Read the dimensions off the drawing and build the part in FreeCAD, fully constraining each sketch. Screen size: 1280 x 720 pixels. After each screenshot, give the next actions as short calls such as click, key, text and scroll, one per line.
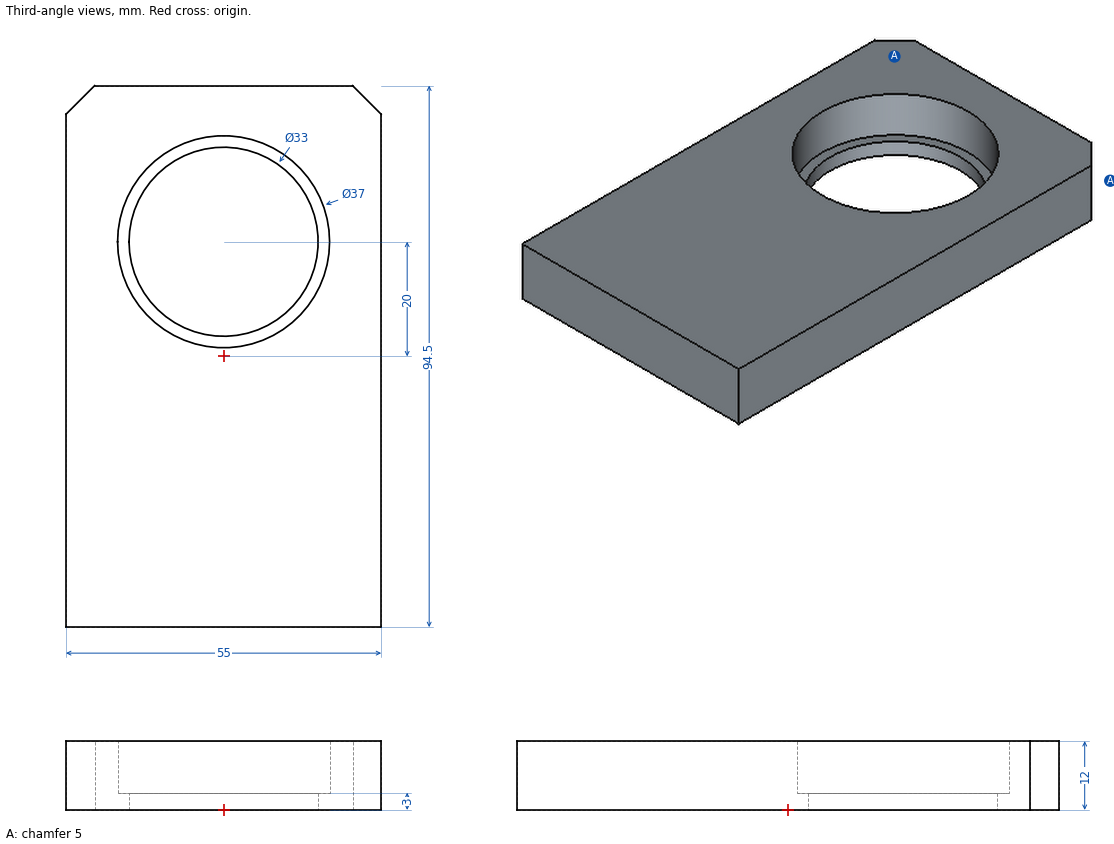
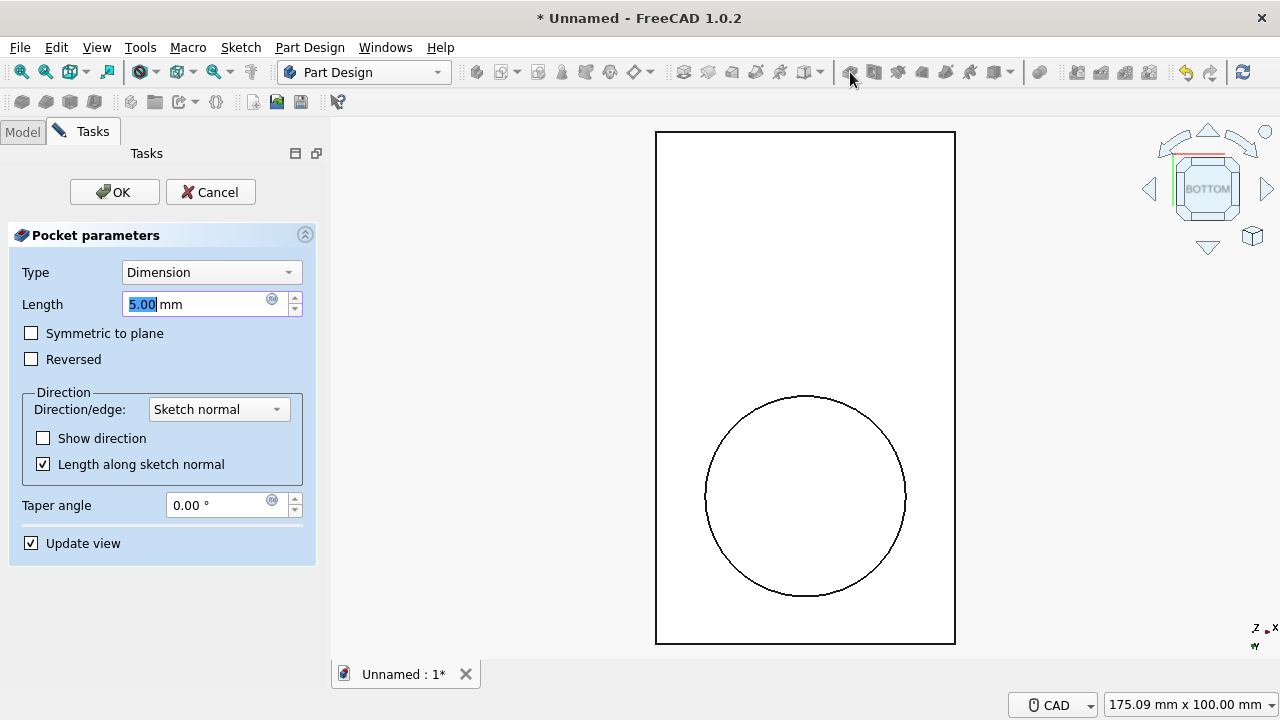
click(212, 272)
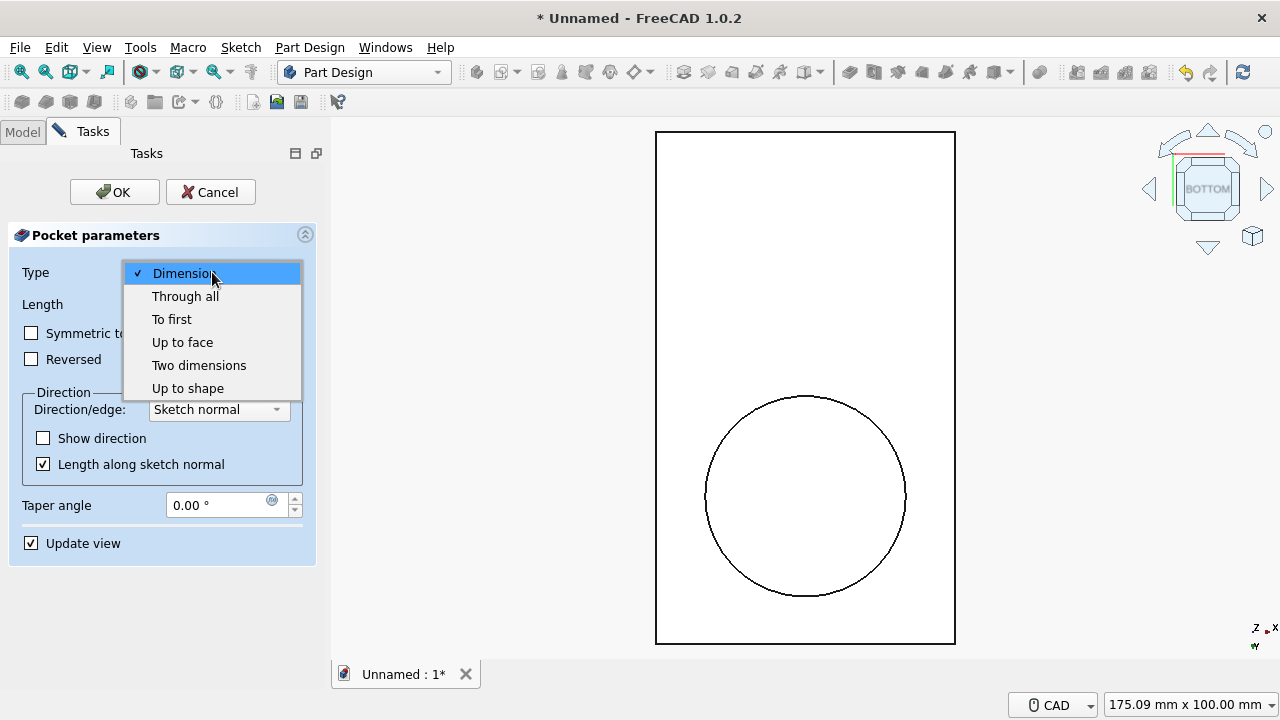
click(212, 320)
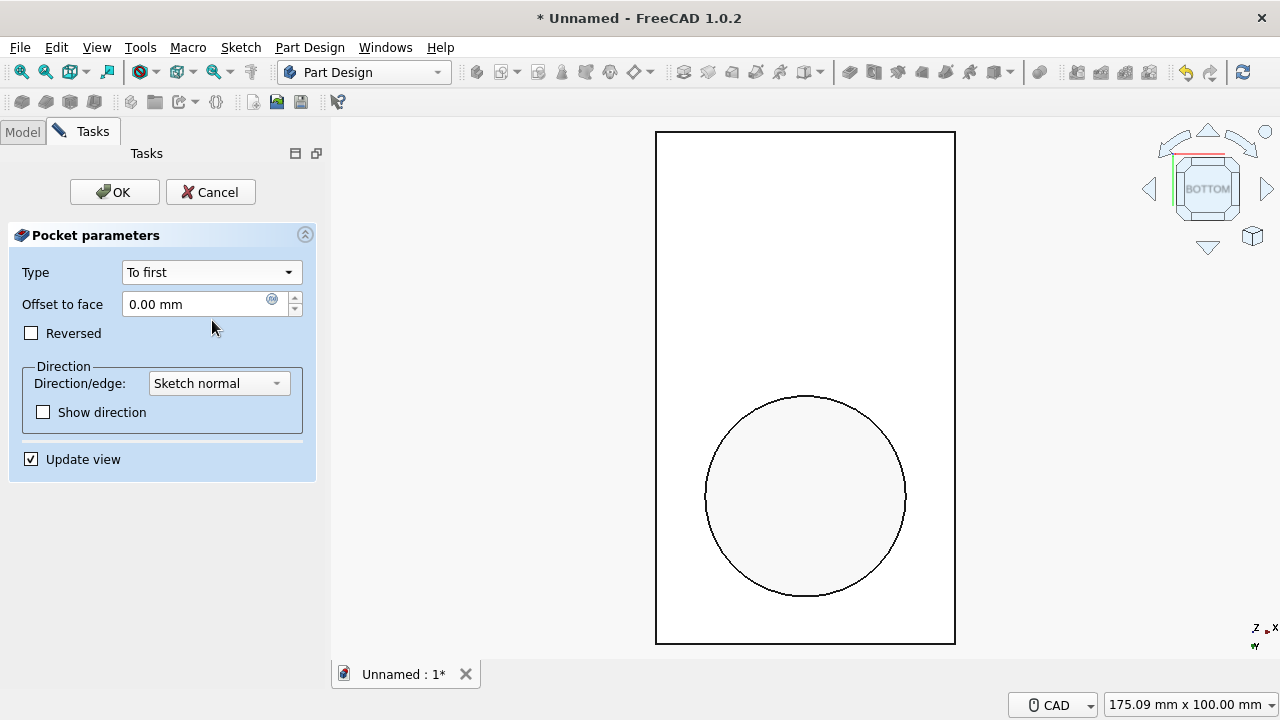
click(115, 192)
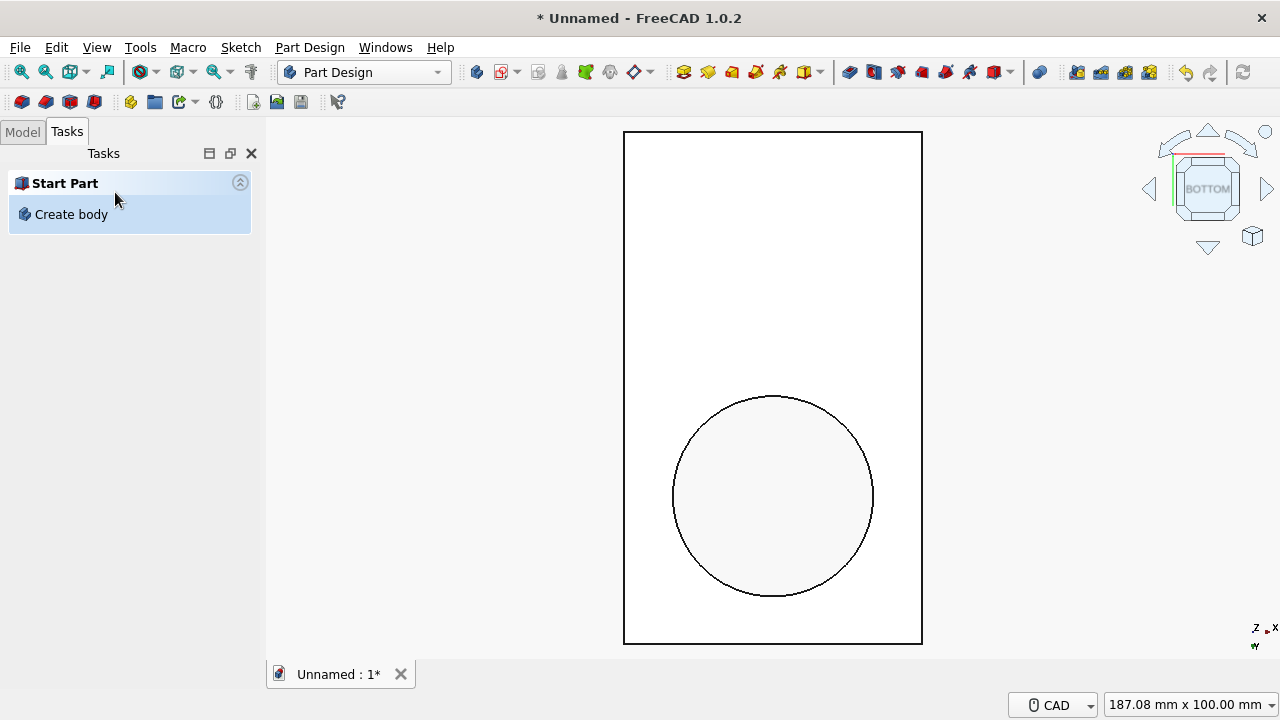
key(0)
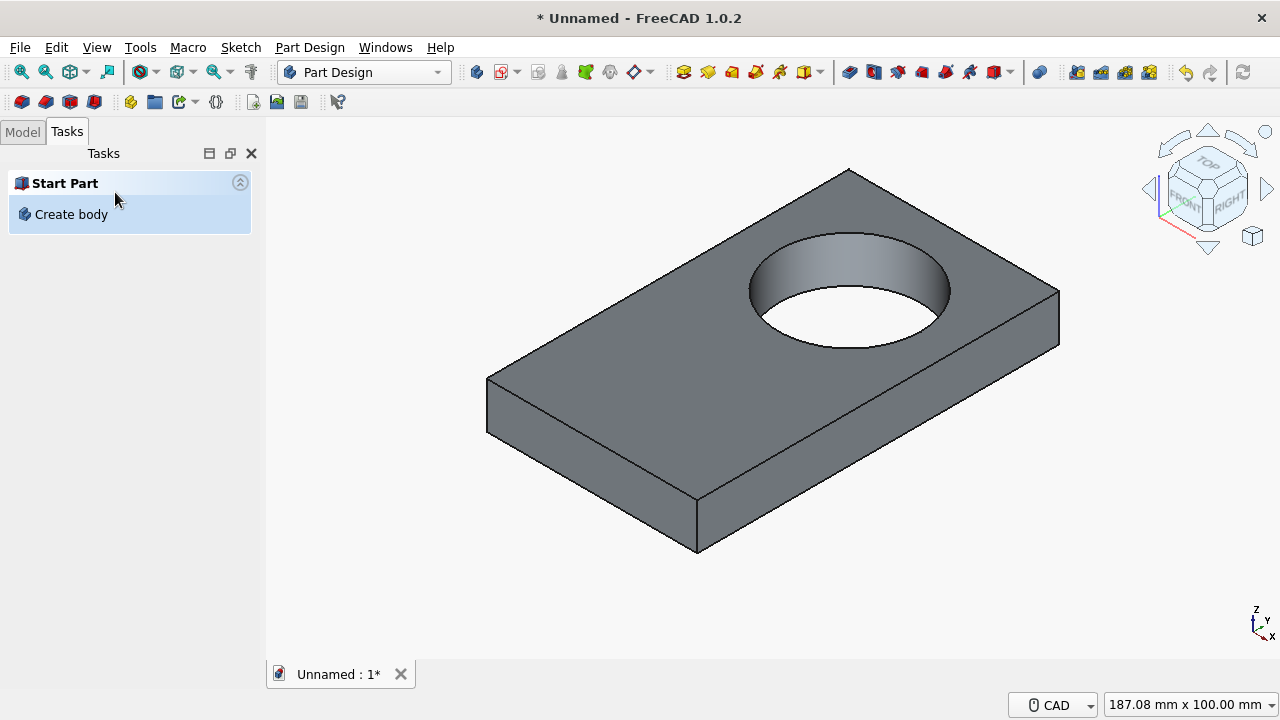
key(2)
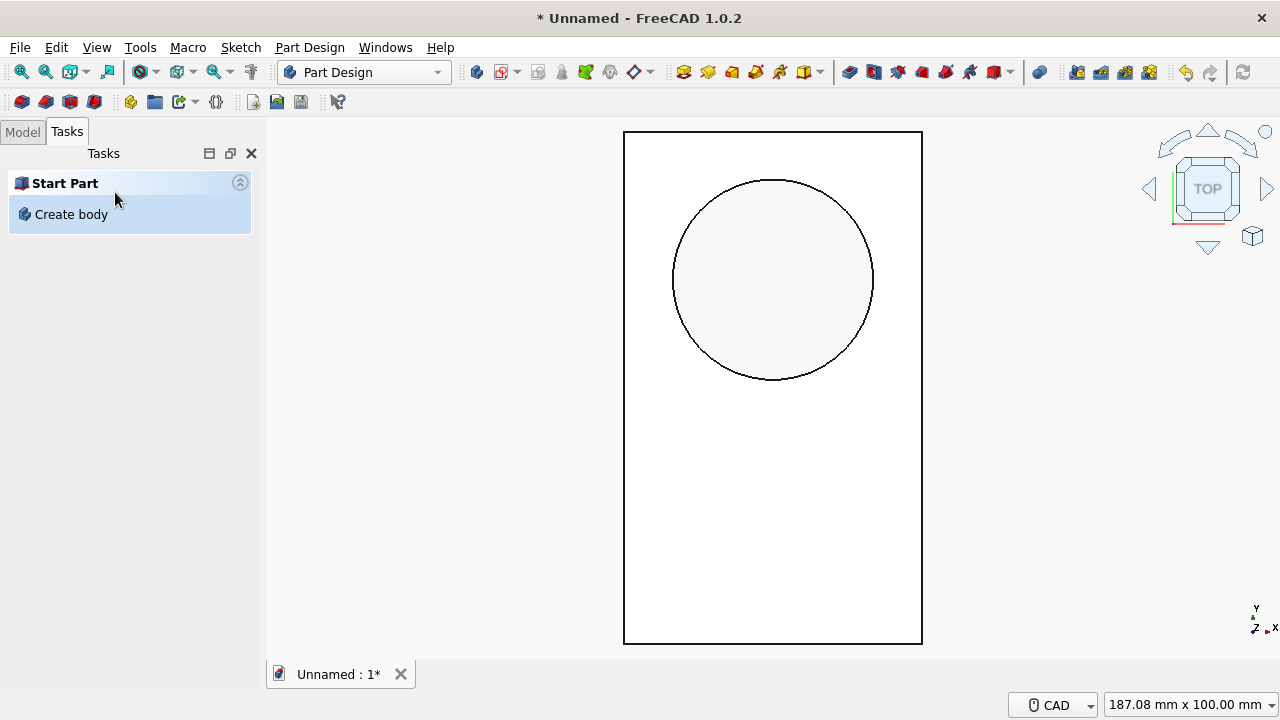
key(1)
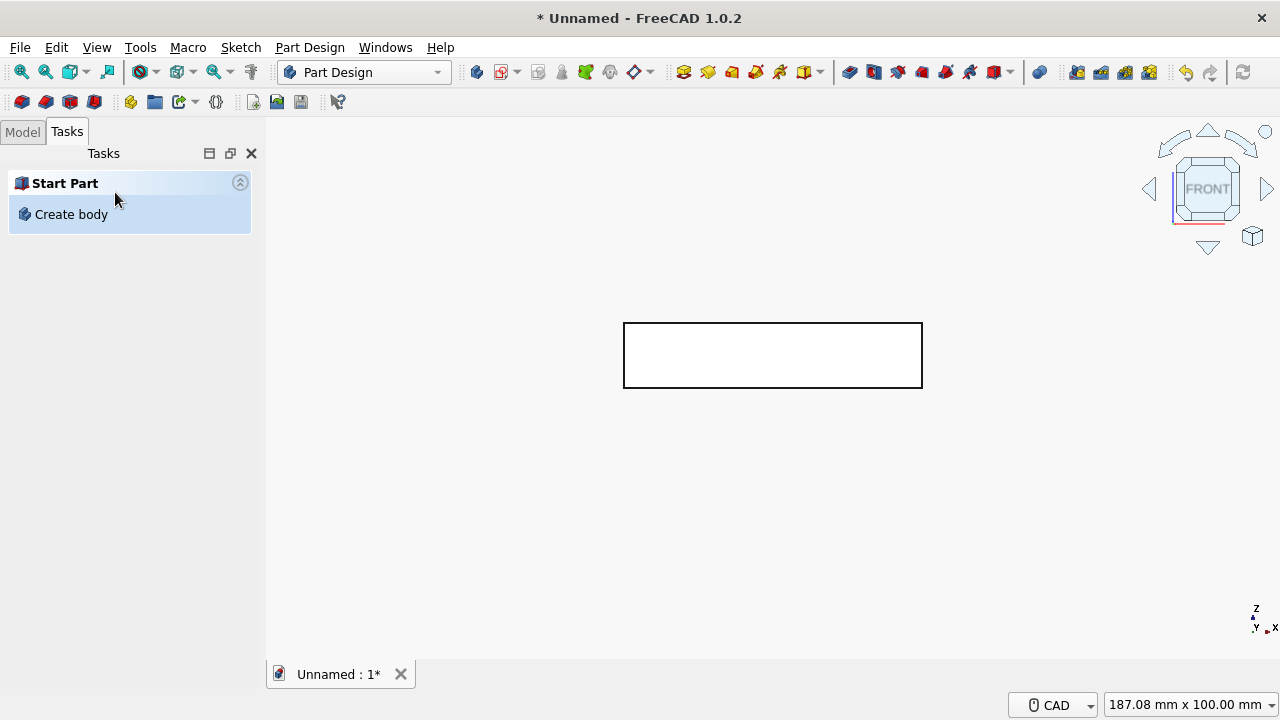
click(22, 72)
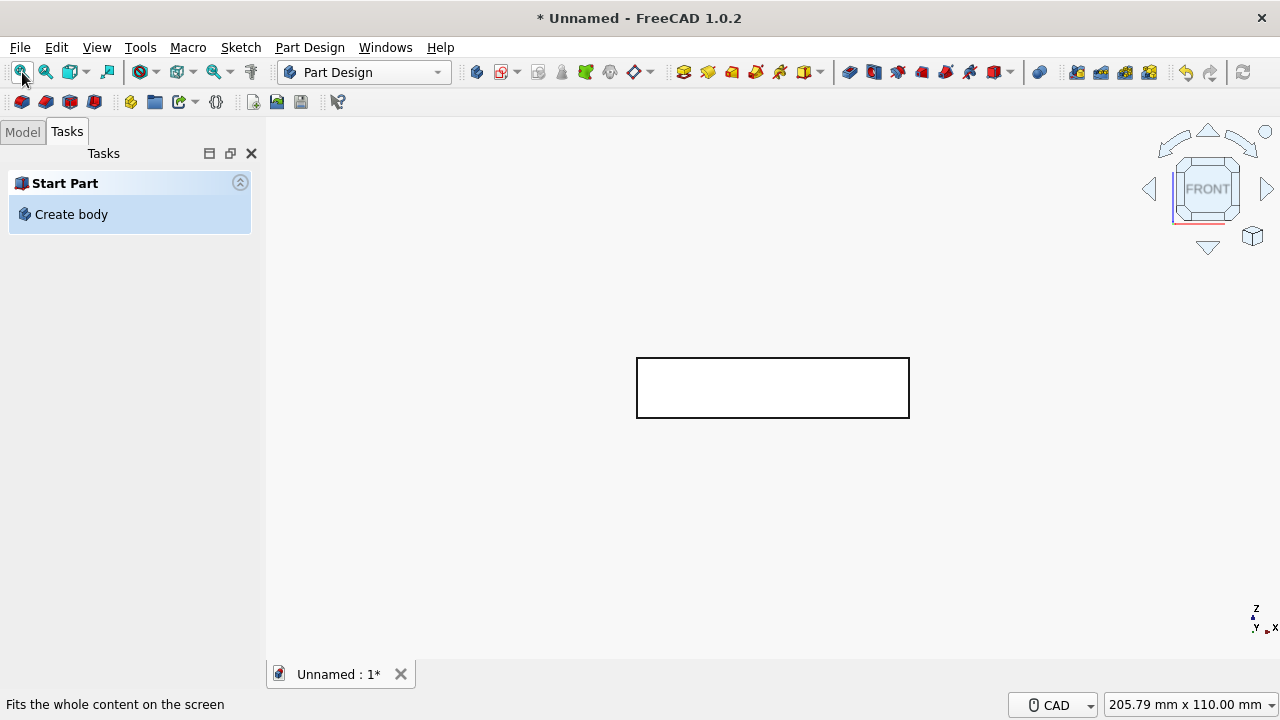
key(3)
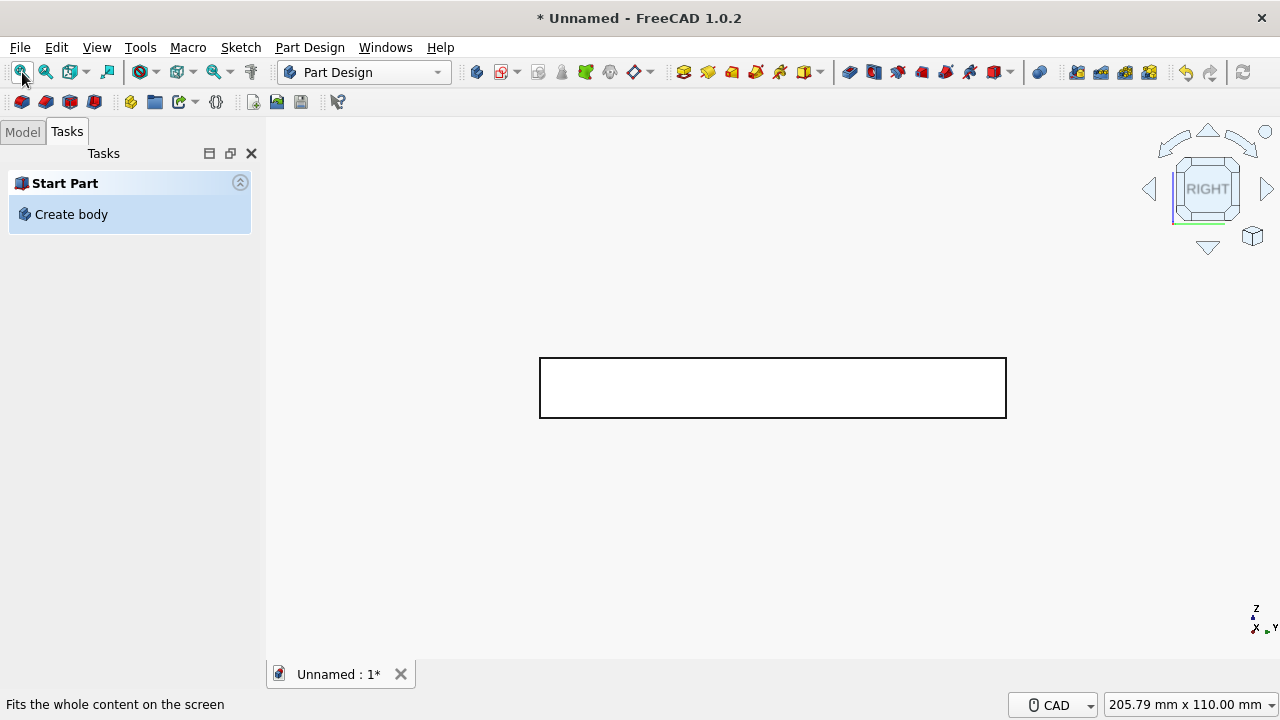
click(1006, 387)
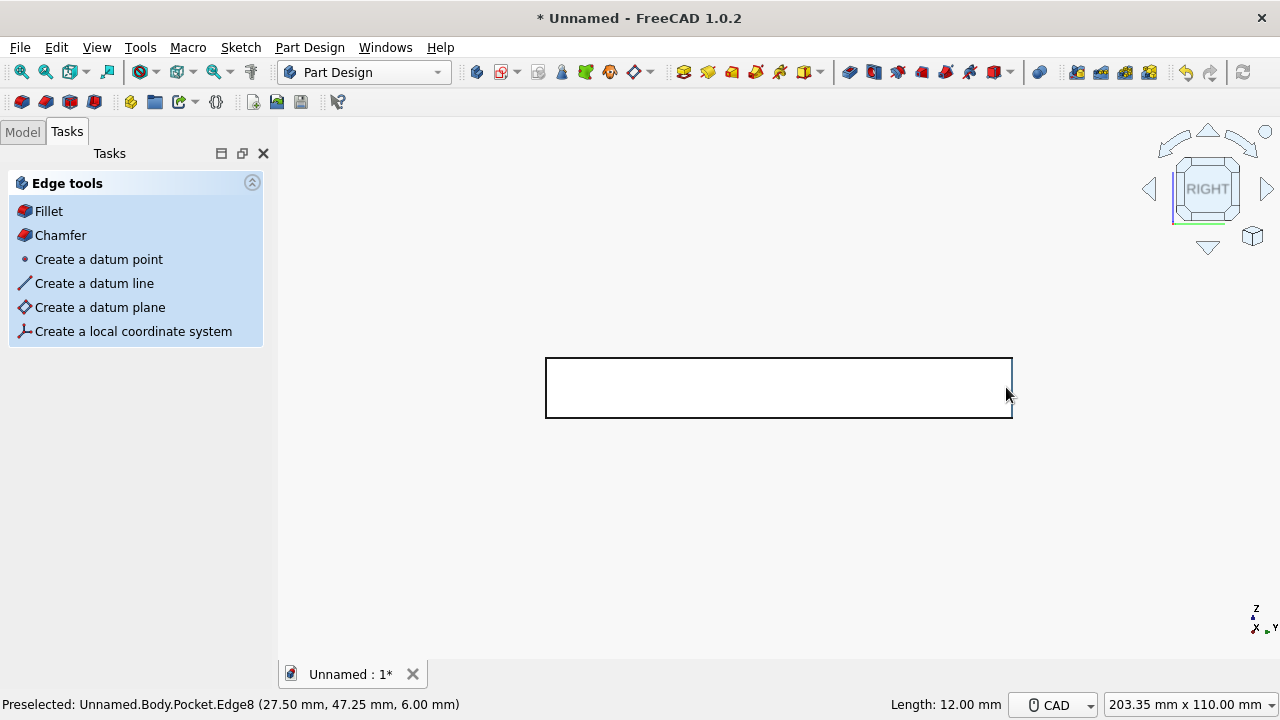
key(5)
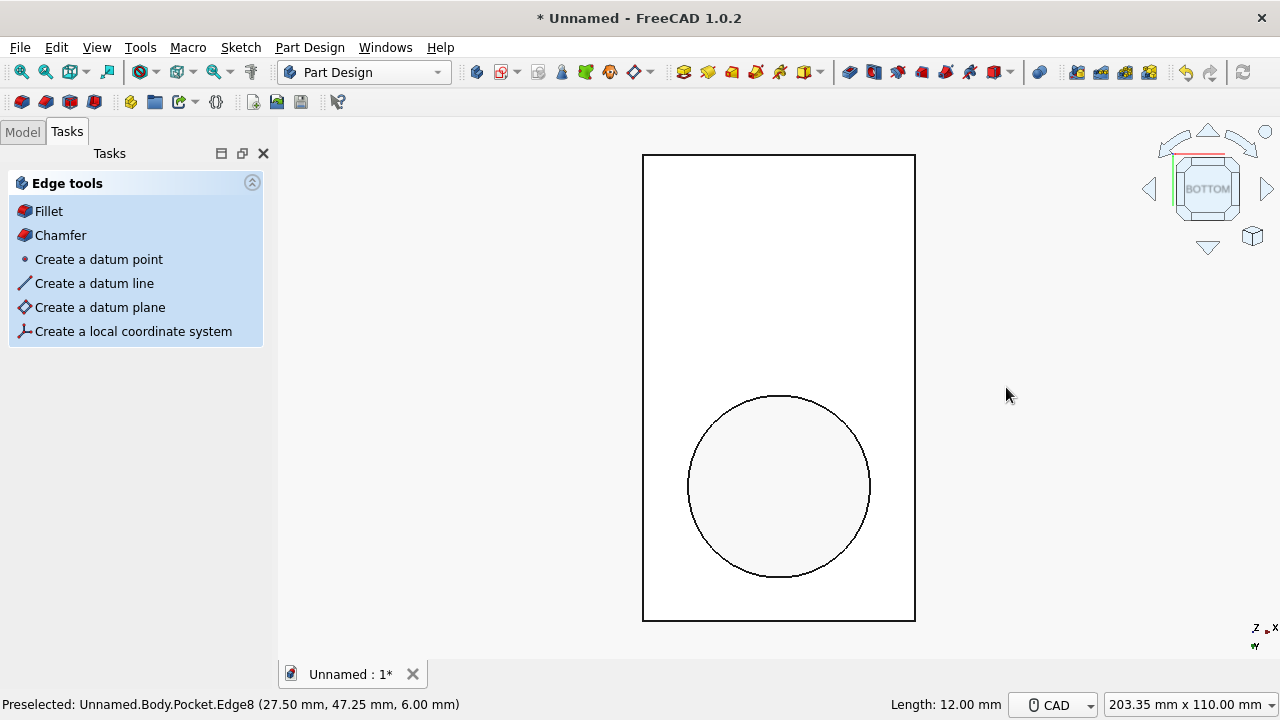
key(4)